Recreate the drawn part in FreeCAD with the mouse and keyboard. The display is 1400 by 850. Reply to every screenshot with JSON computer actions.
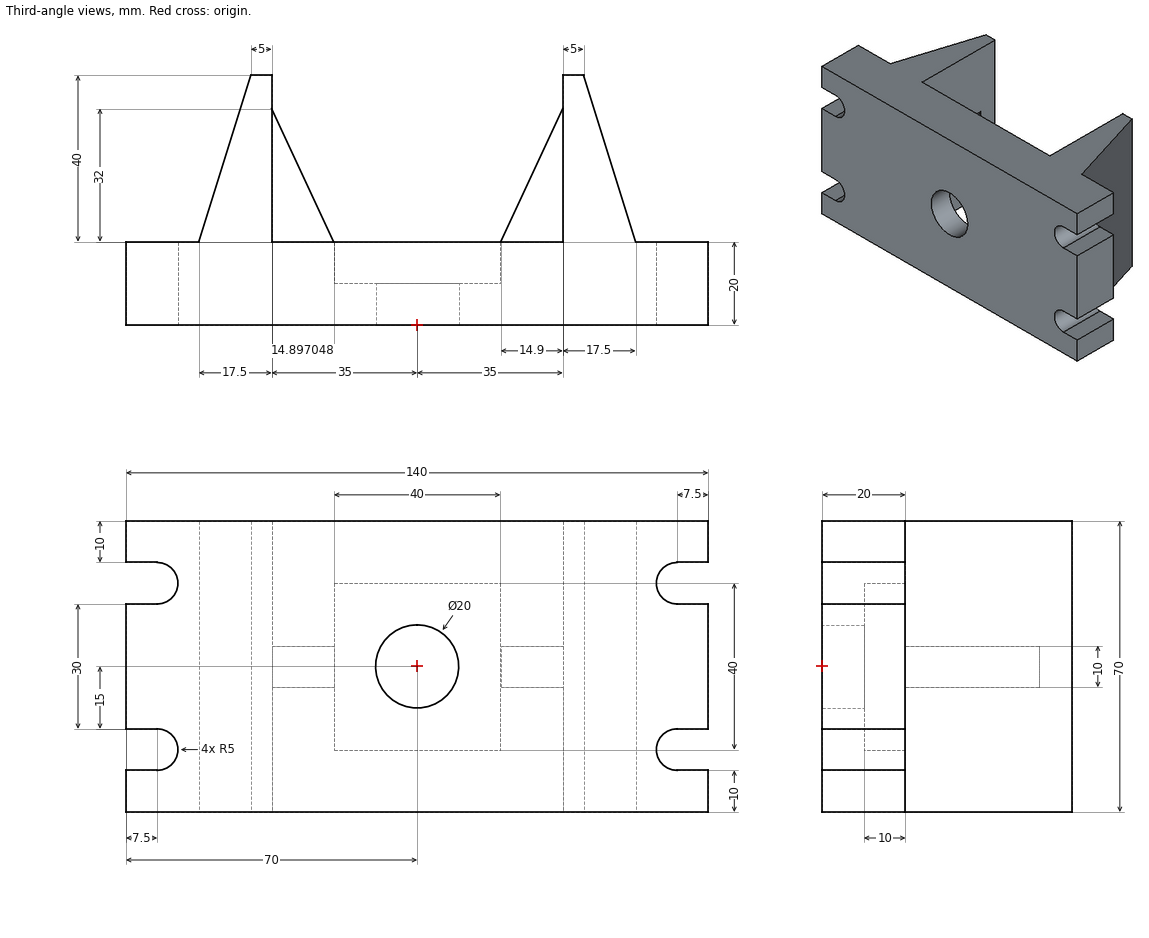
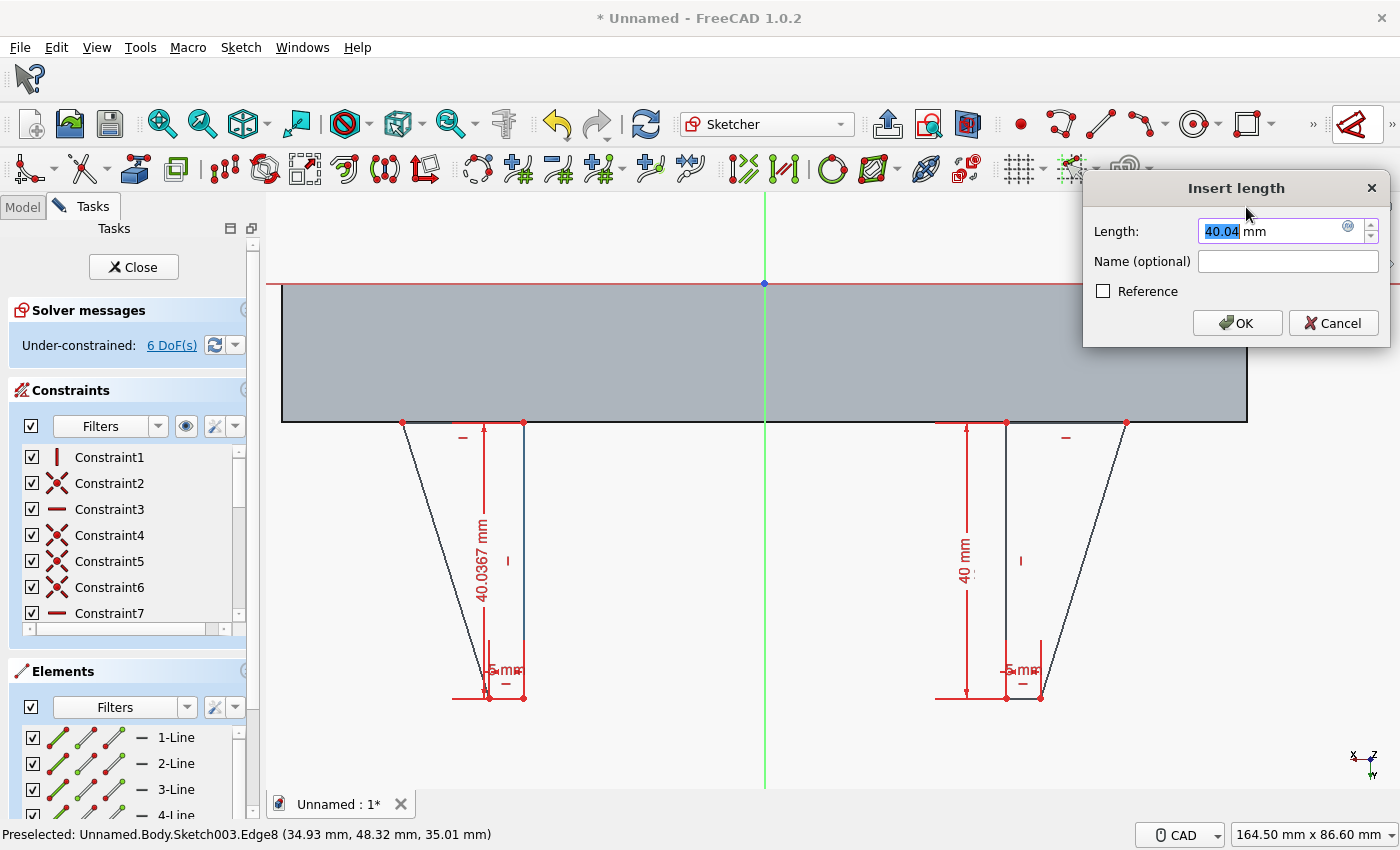
{"action": "type", "text": "40"}
{"action": "key", "text": "Return"}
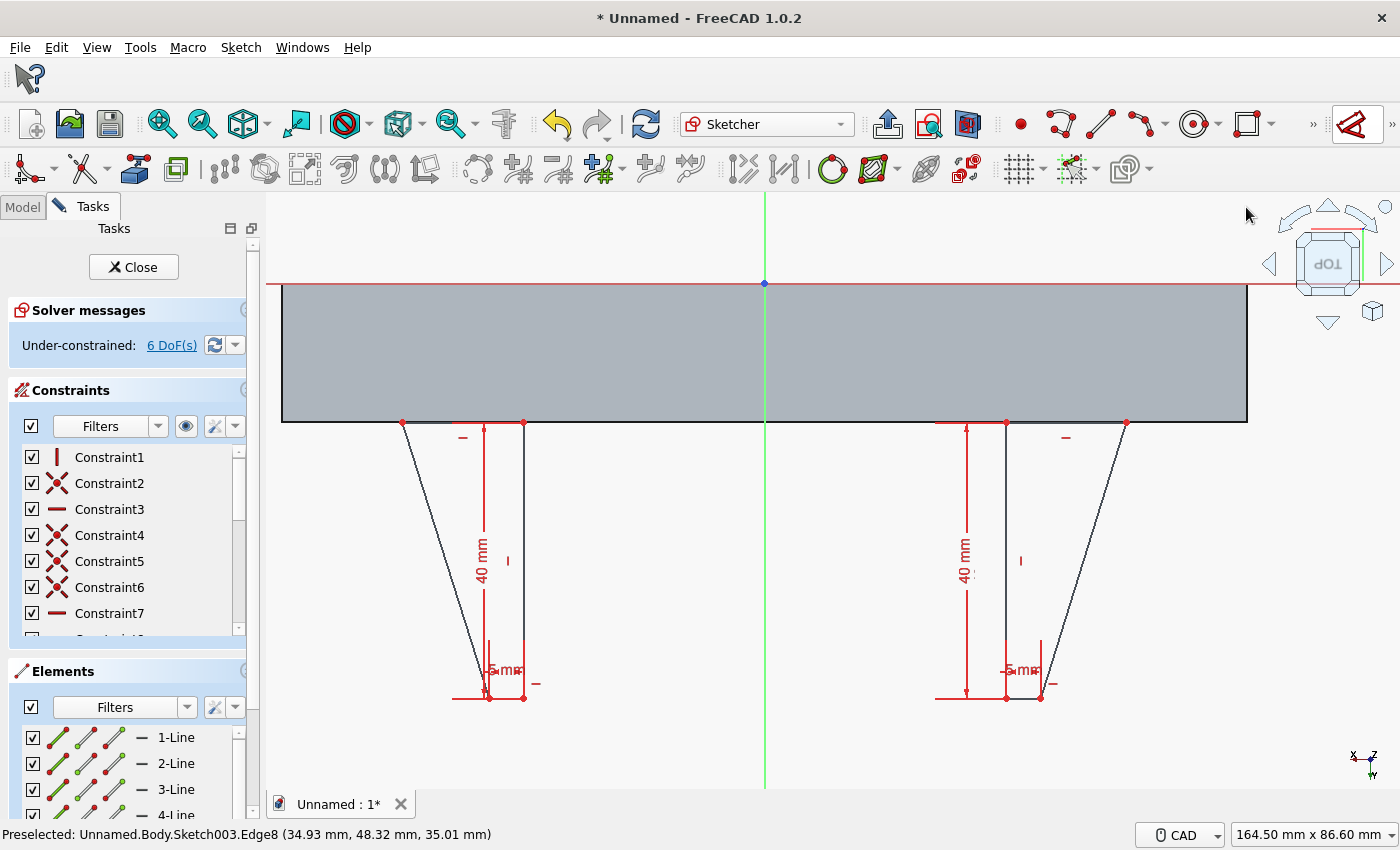
{"action": "left_click", "coordinate": [1006, 423]}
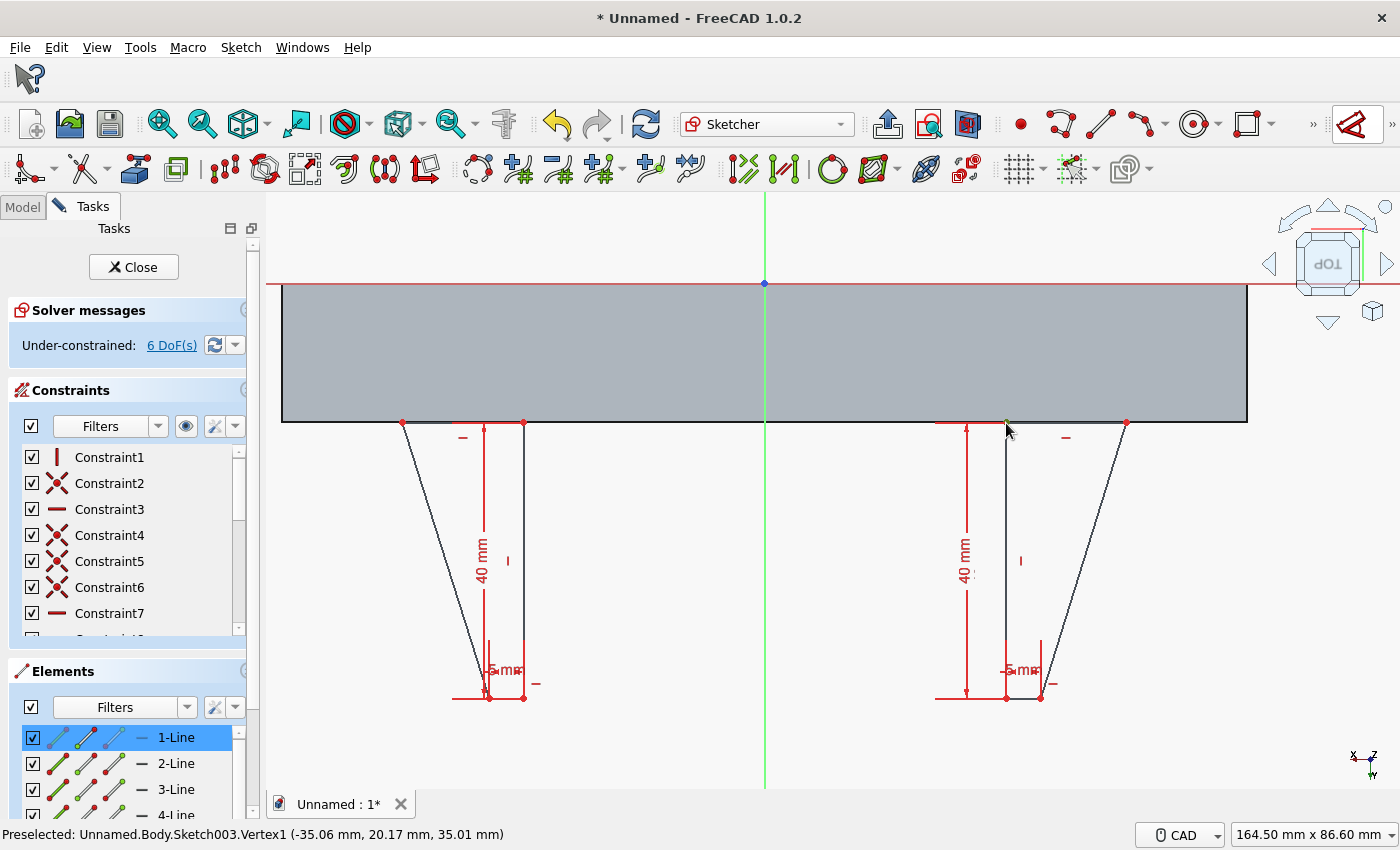
{"action": "key", "text": "l"}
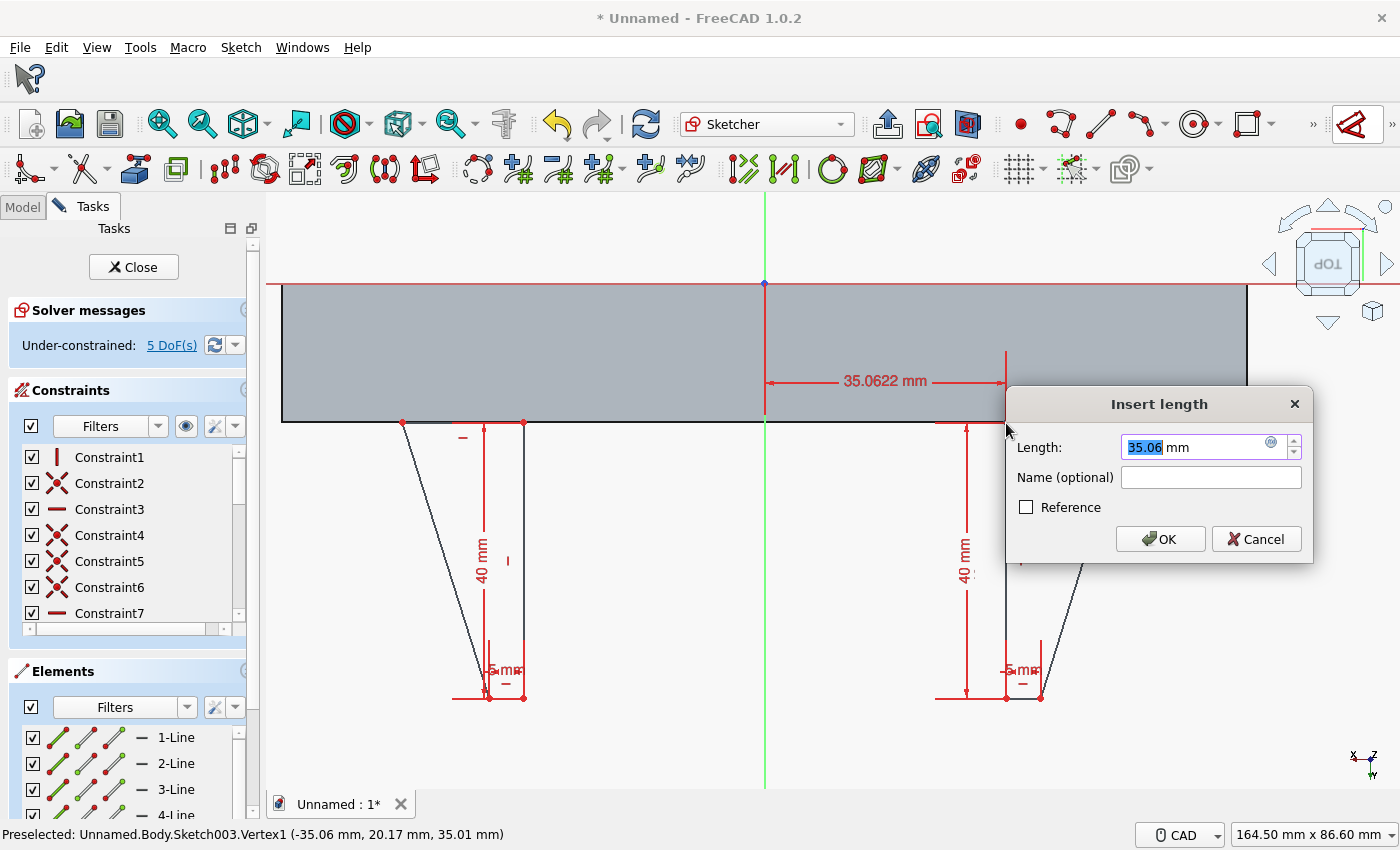
{"action": "type", "text": "35"}
{"action": "key", "text": "Return"}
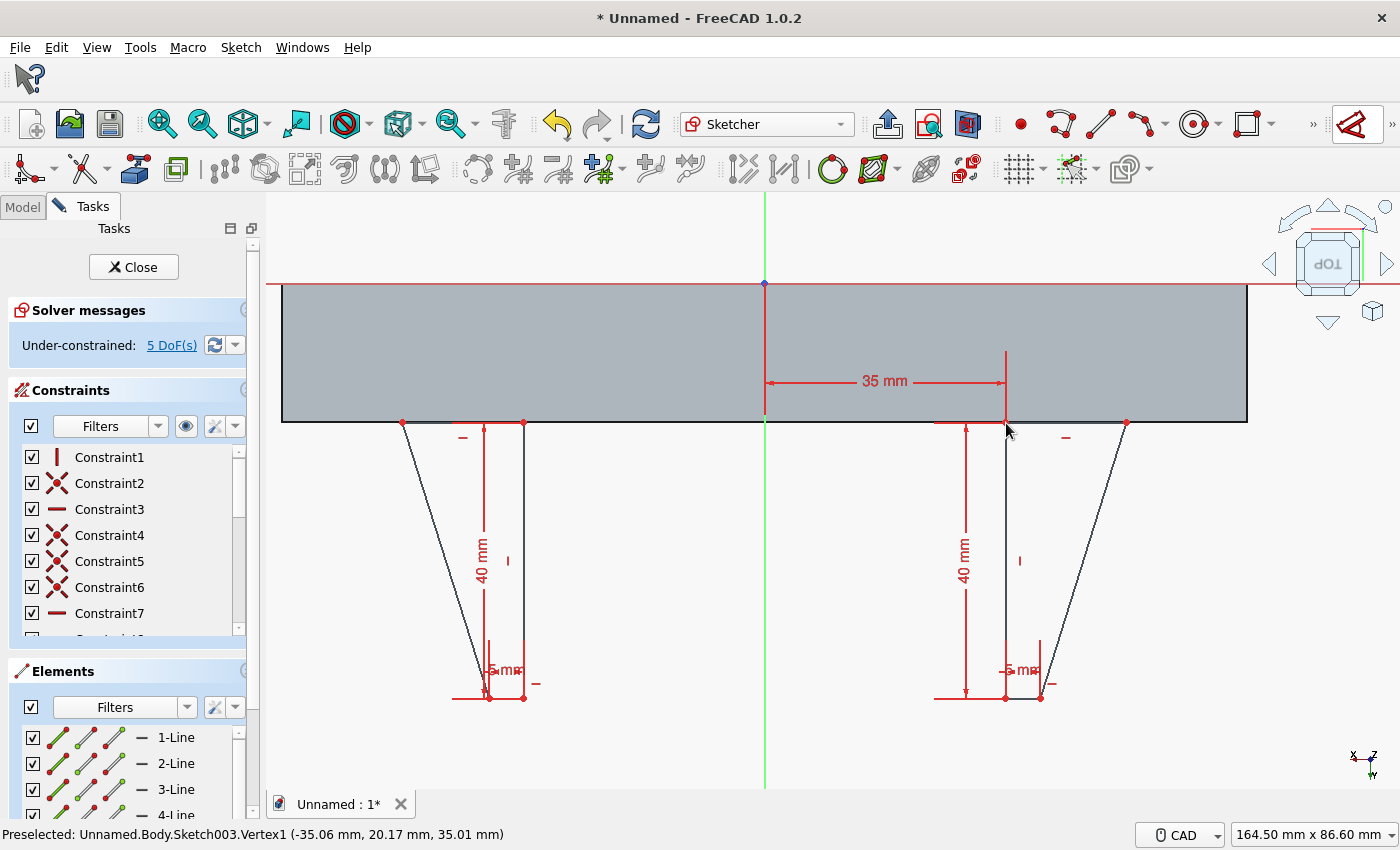
{"action": "left_click", "coordinate": [1006, 423]}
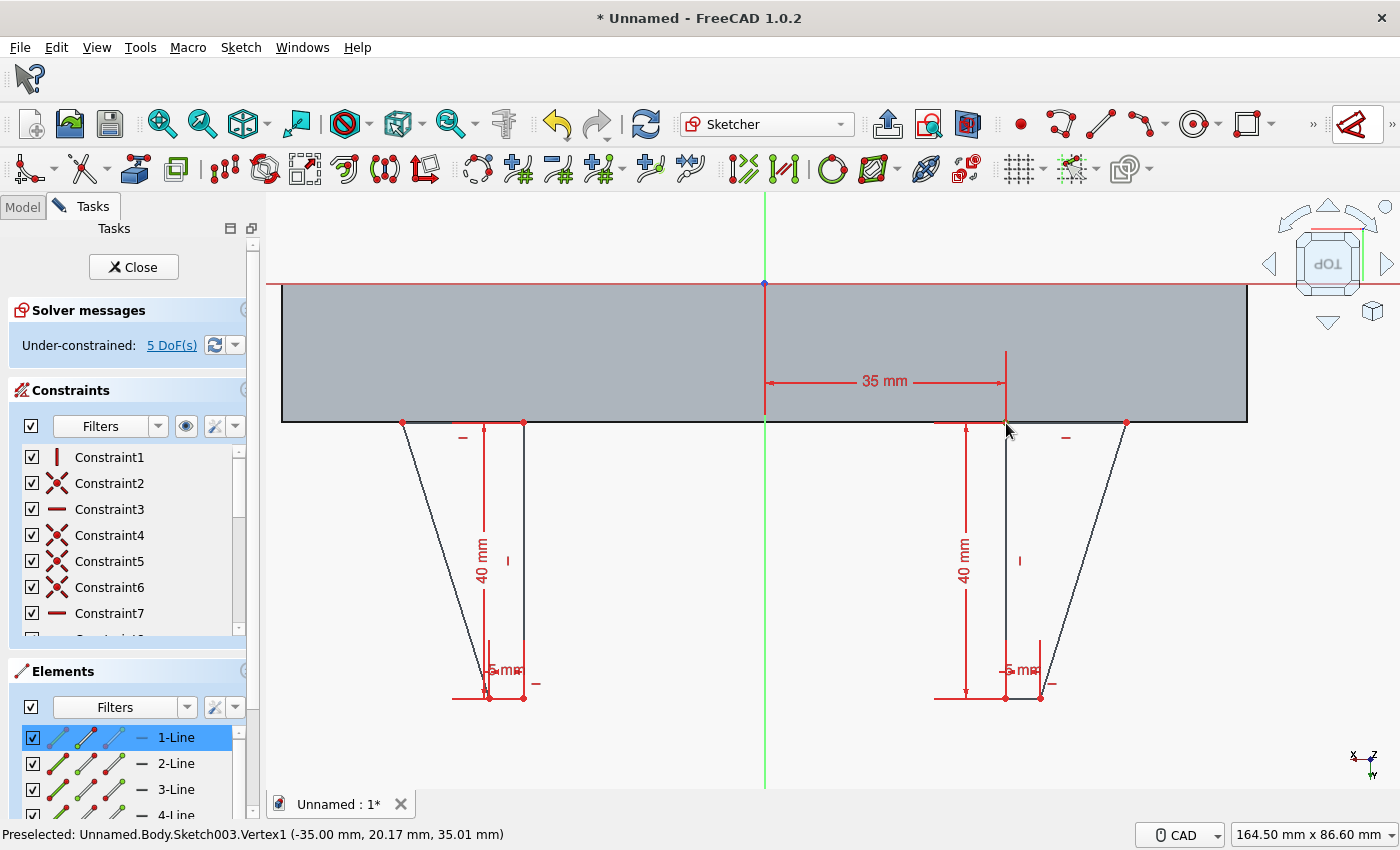
{"action": "left_click", "coordinate": [1378, 124]}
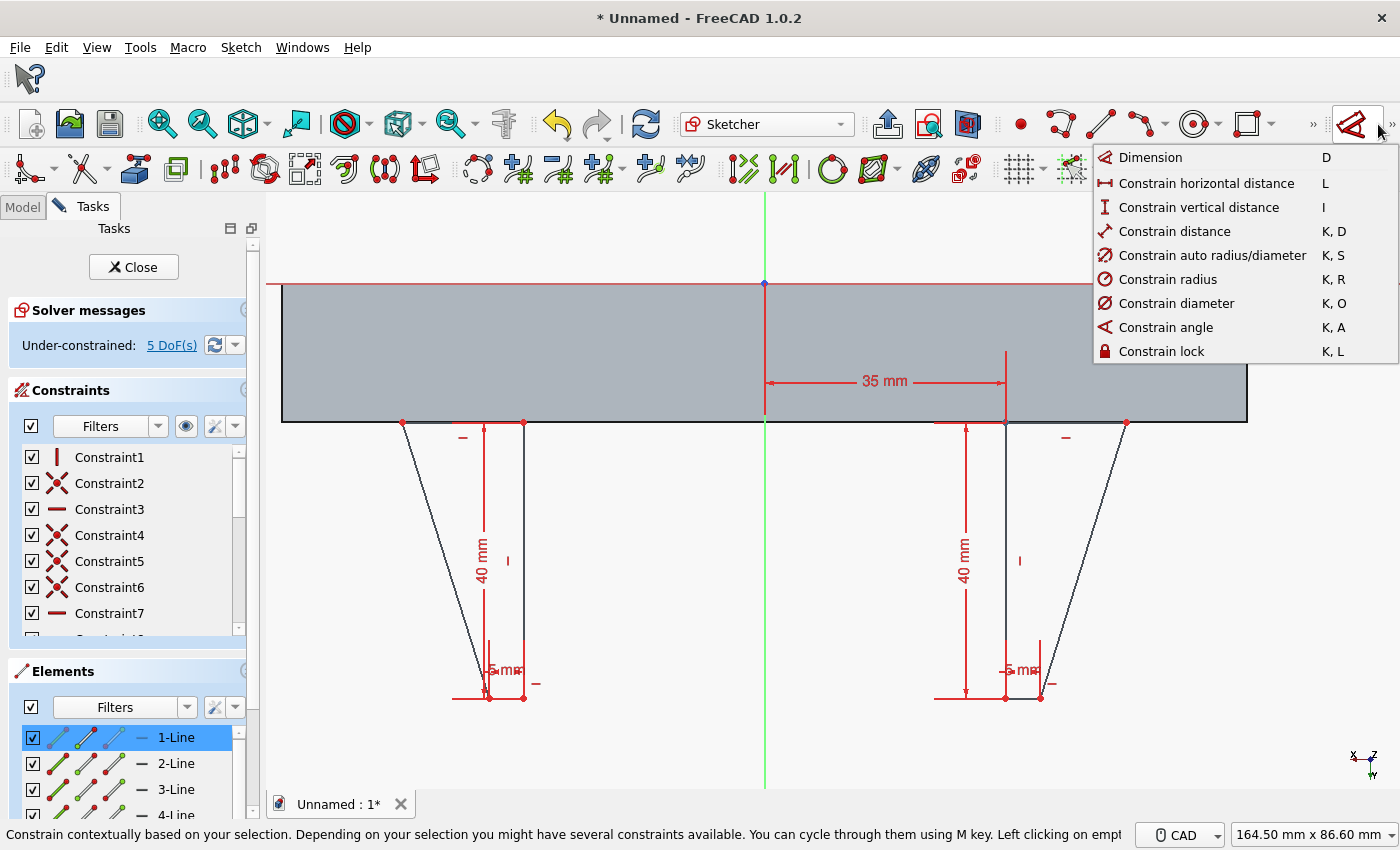
{"action": "left_click", "coordinate": [1246, 207]}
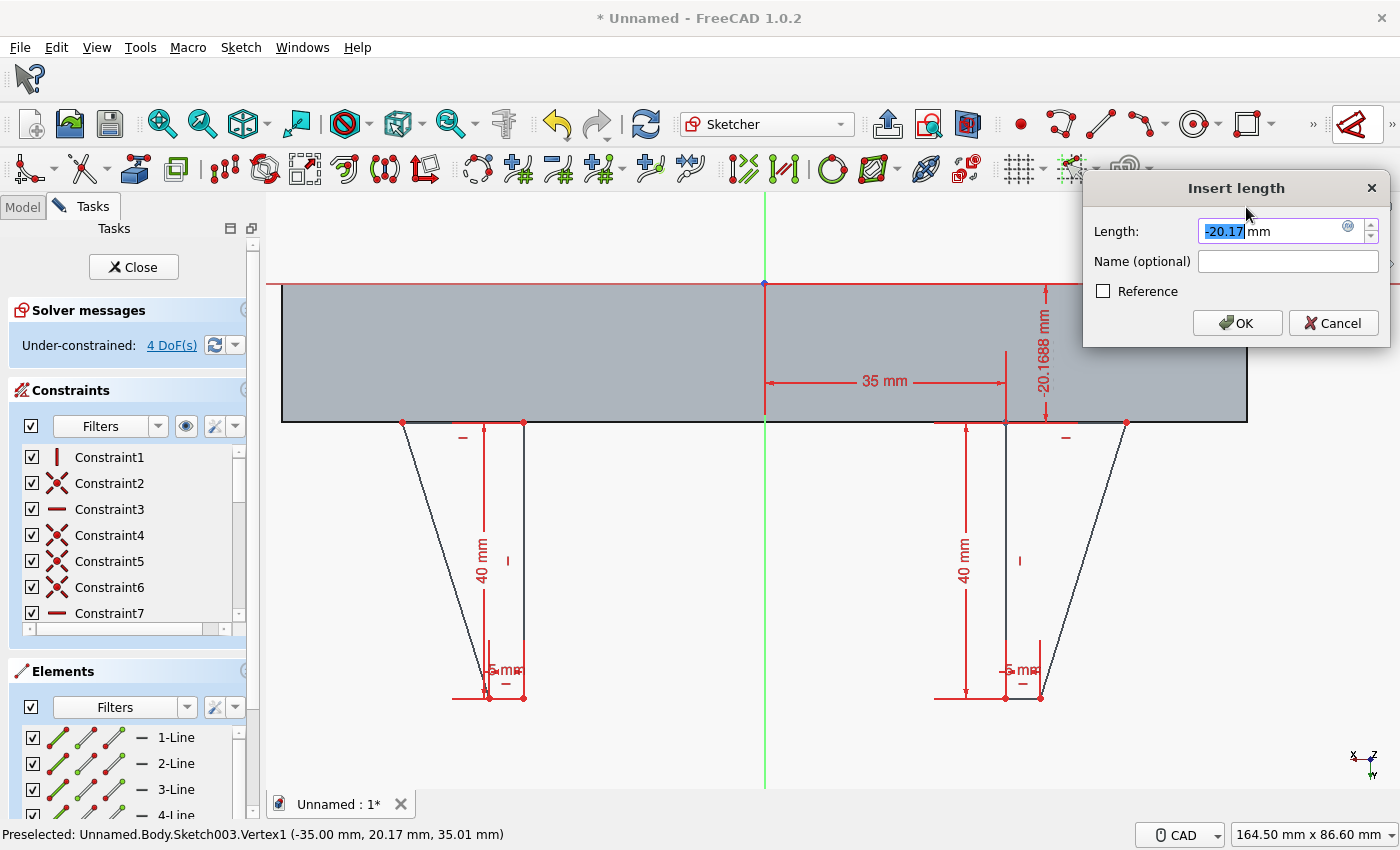
{"action": "type", "text": "-20"}
{"action": "key", "text": "Return"}